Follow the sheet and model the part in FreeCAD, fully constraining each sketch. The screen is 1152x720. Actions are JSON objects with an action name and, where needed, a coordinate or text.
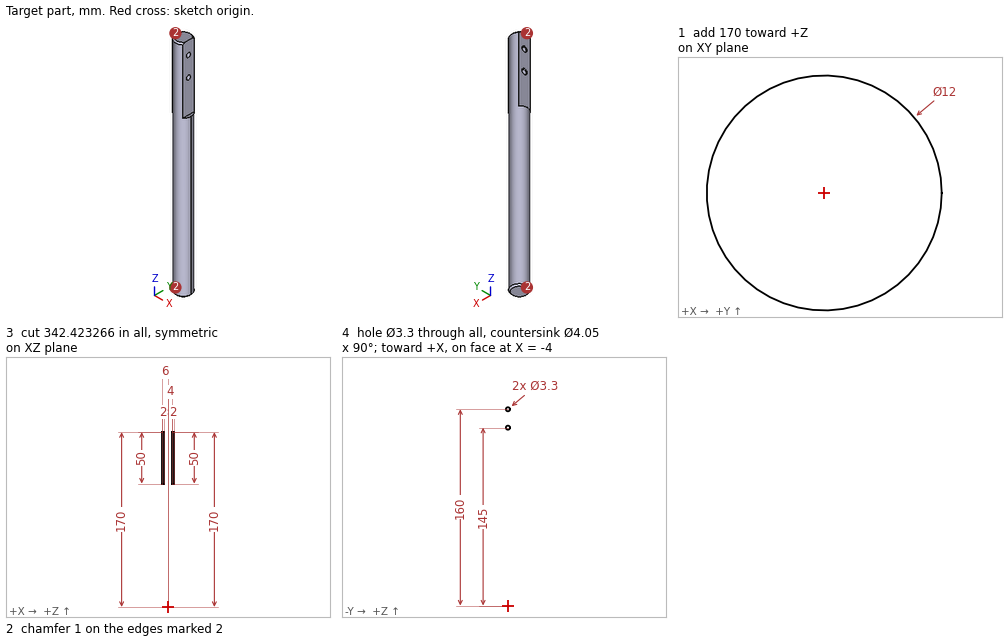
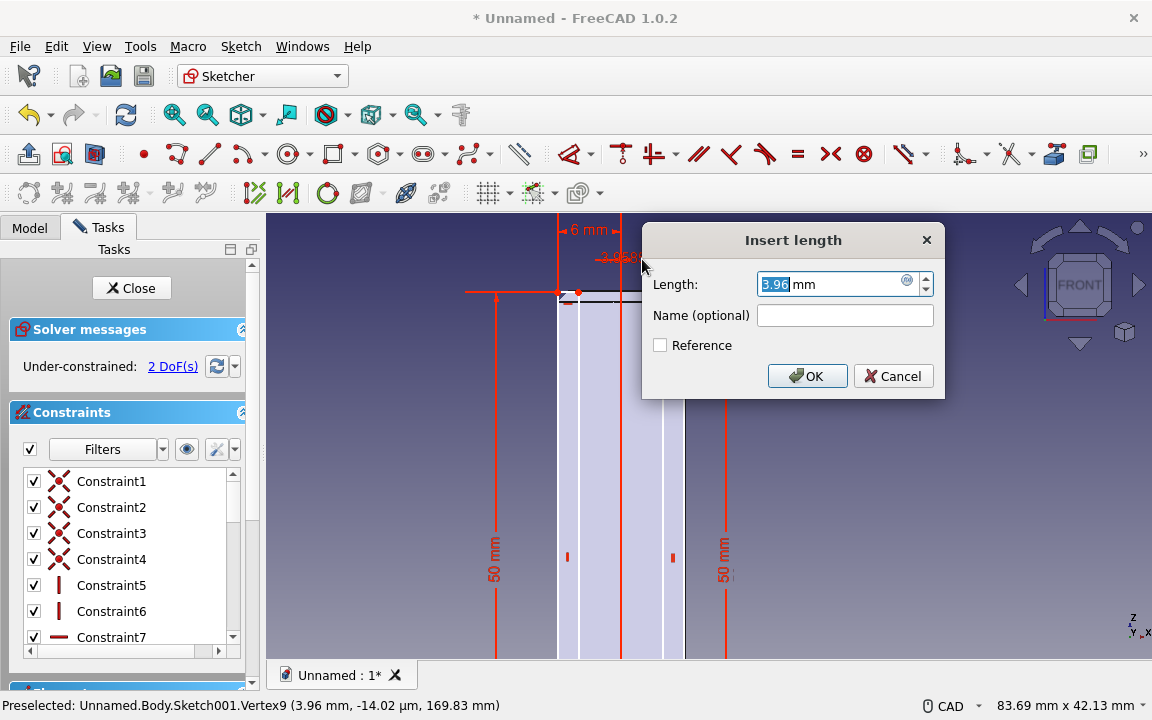
{"action": "type", "text": "4"}
{"action": "key", "text": "Return"}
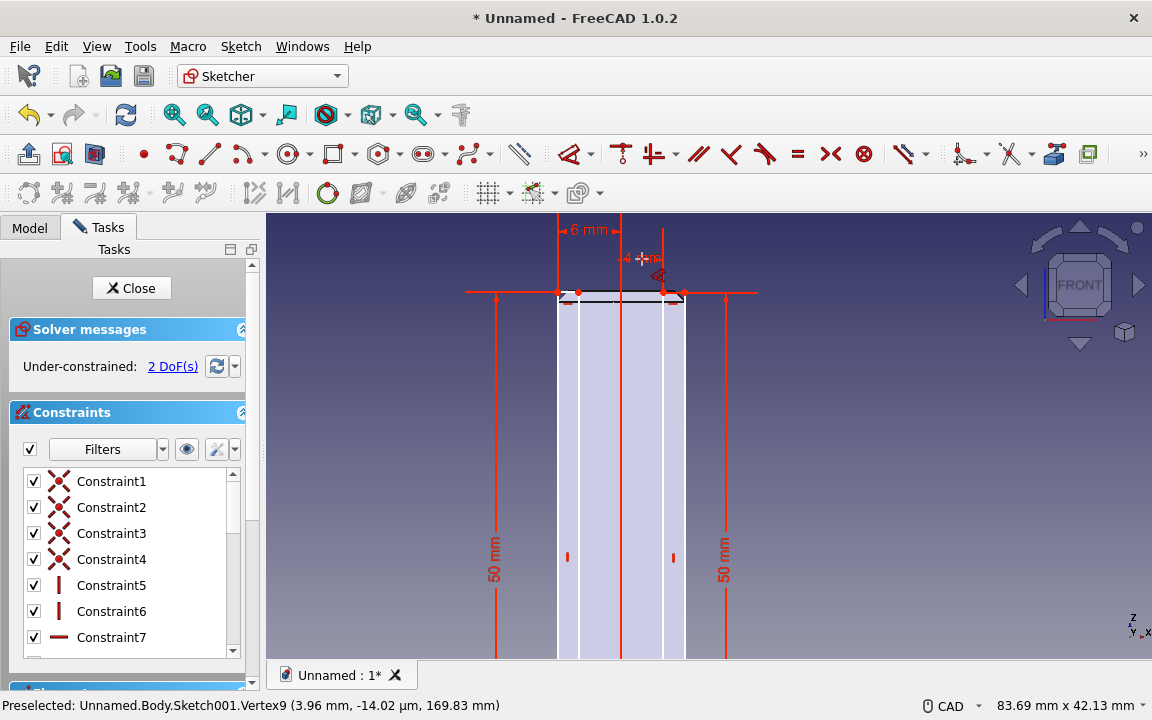
{"action": "left_click", "coordinate": [558, 292]}
{"action": "left_click", "coordinate": [524, 462]}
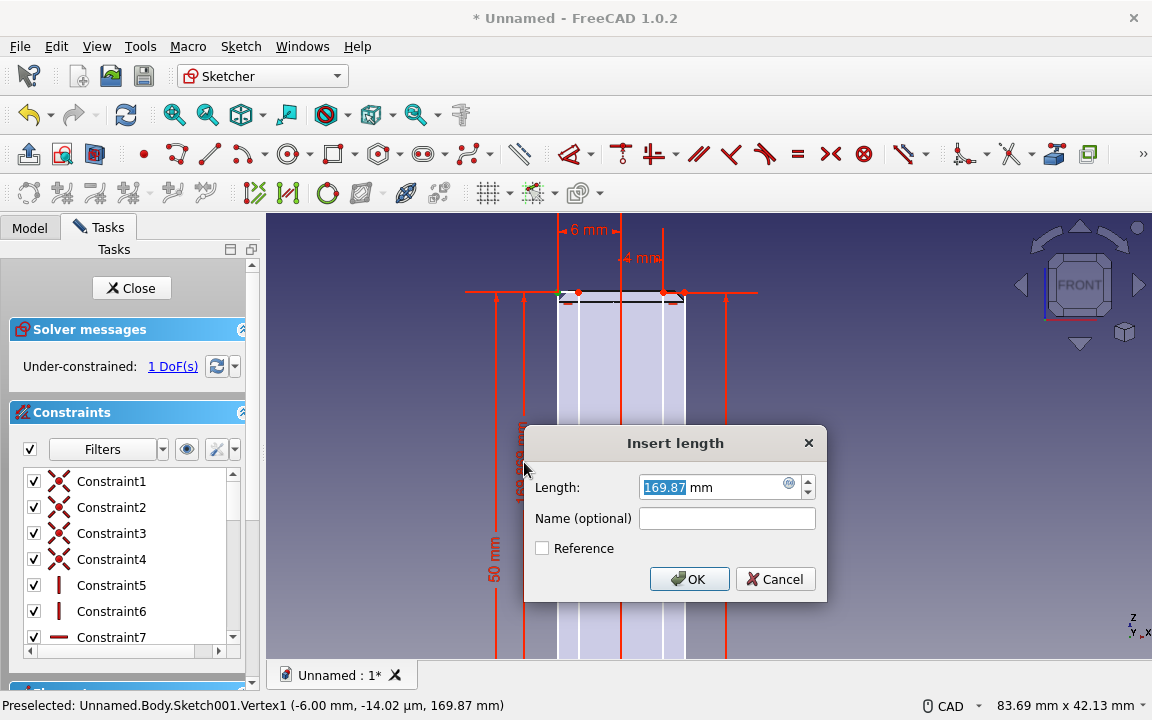
{"action": "type", "text": "170"}
{"action": "key", "text": "Return"}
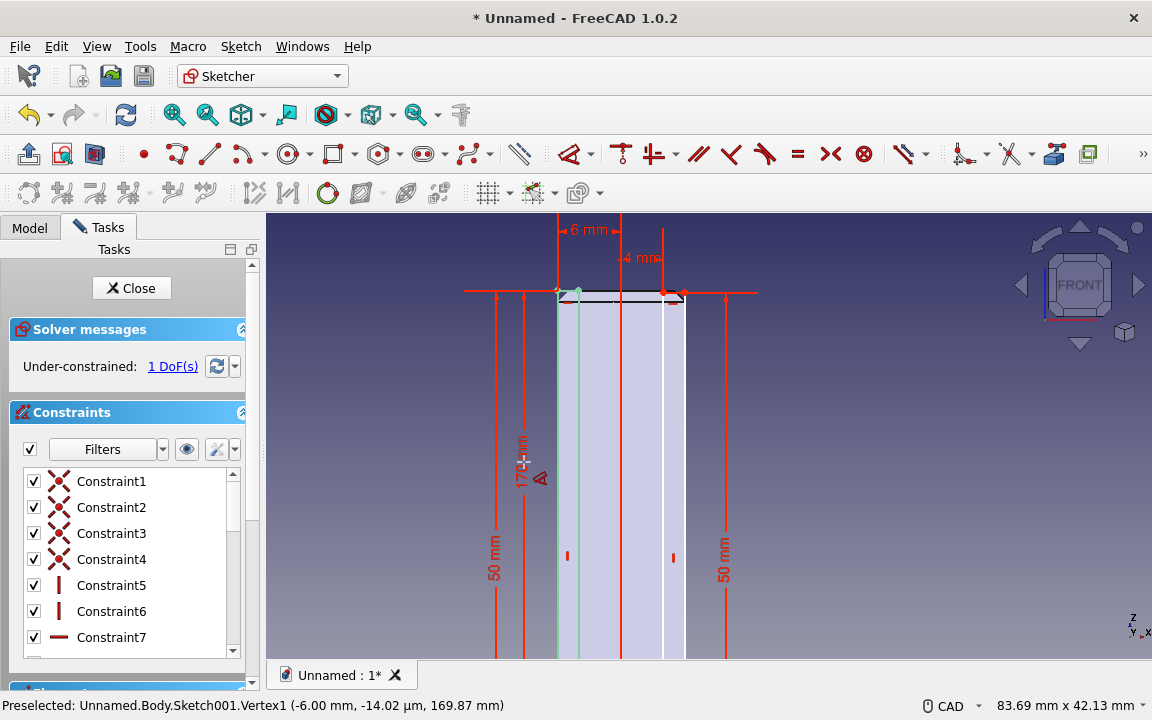
{"action": "left_click", "coordinate": [663, 293]}
{"action": "left_click", "coordinate": [721, 462]}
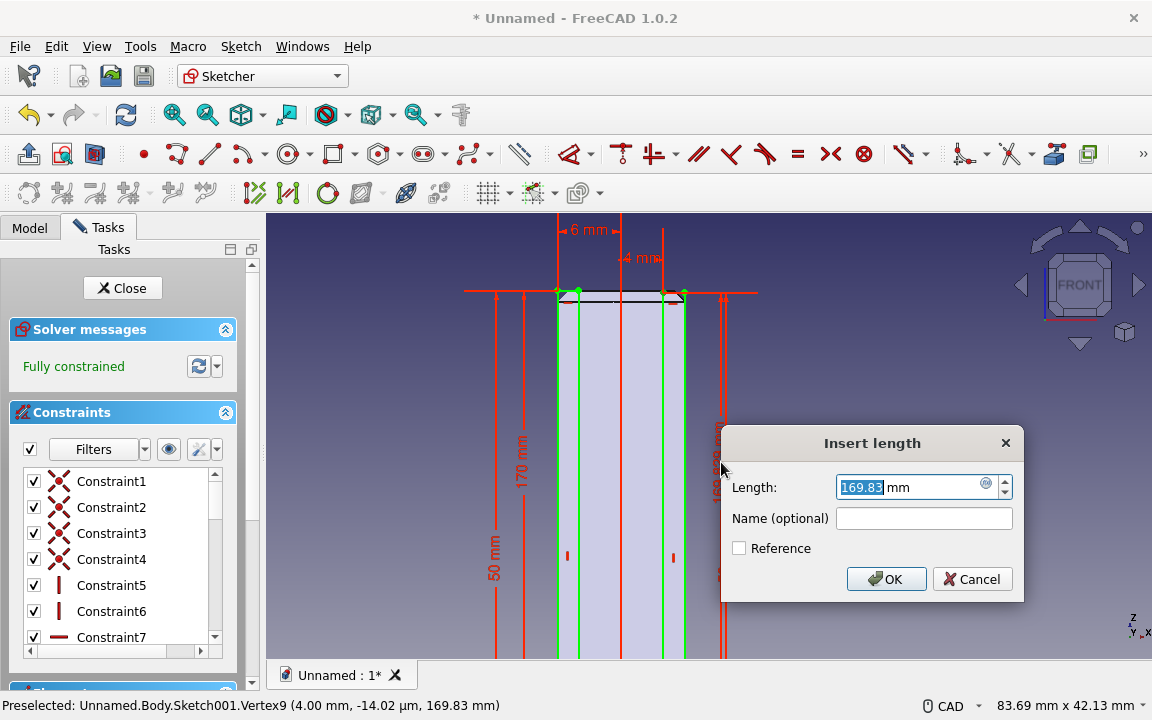
{"action": "type", "text": "170"}
{"action": "key", "text": "Return"}
{"action": "key", "text": "Escape"}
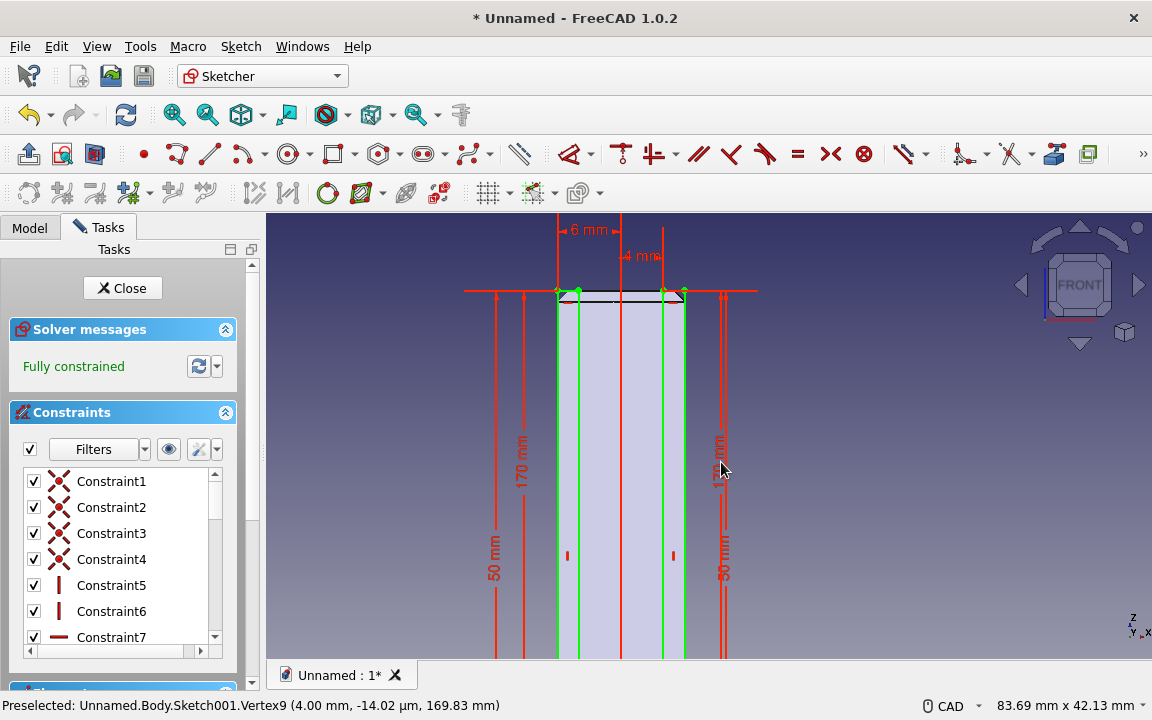
{"action": "left_click", "coordinate": [123, 288]}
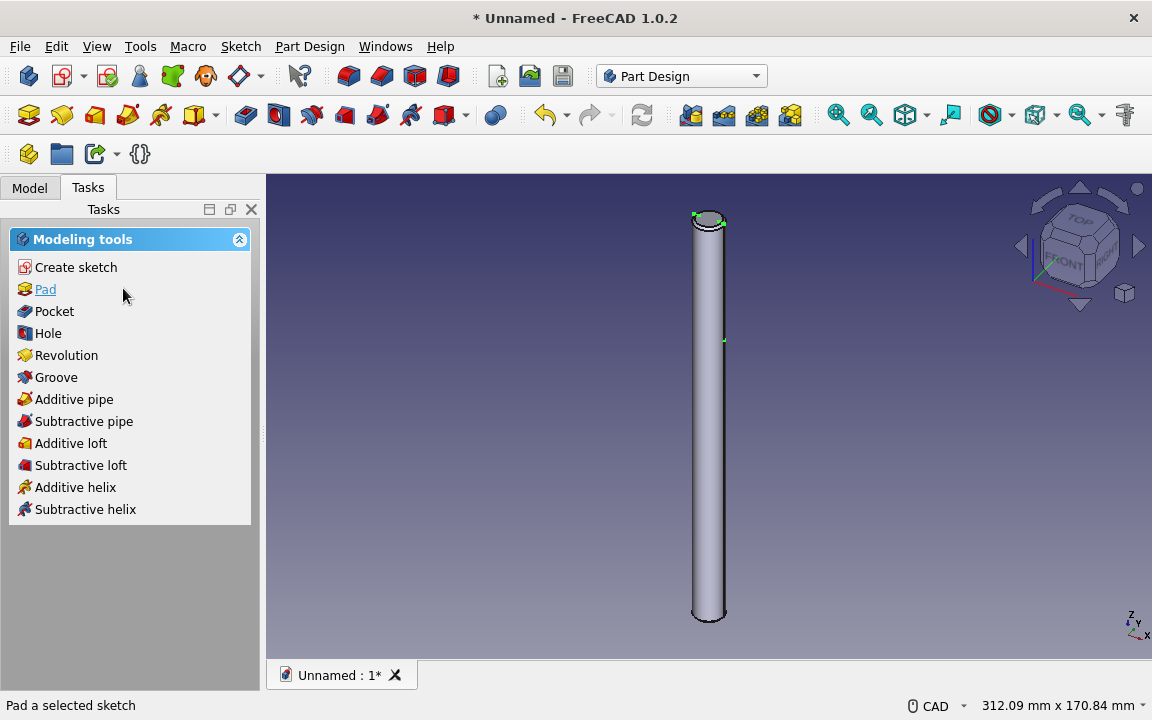
{"action": "left_click", "coordinate": [246, 116]}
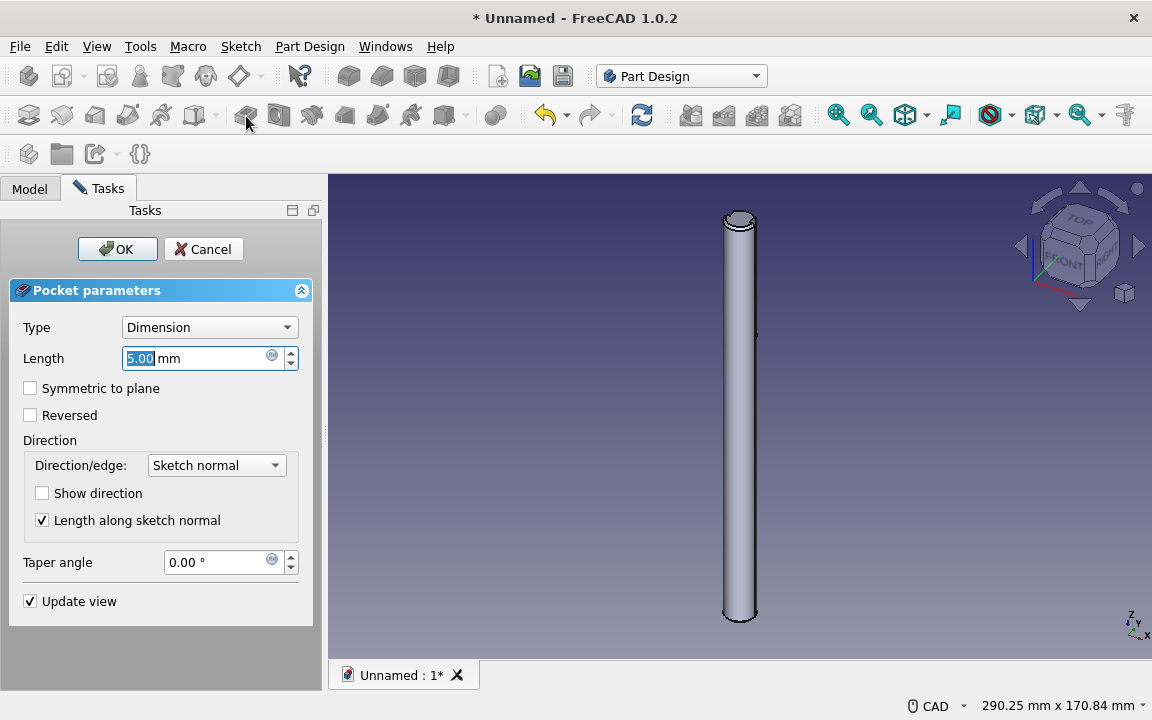
{"action": "type", "text": "342.423266"}
{"action": "key", "text": "Tab"}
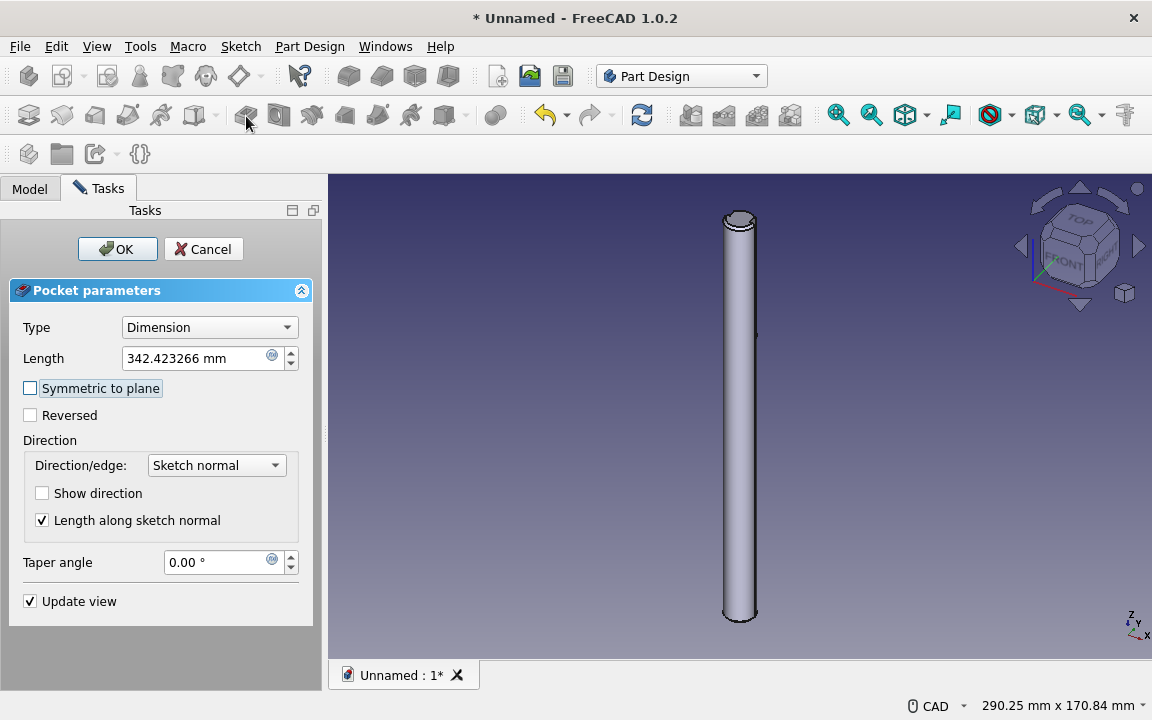
{"action": "left_click", "coordinate": [31, 388]}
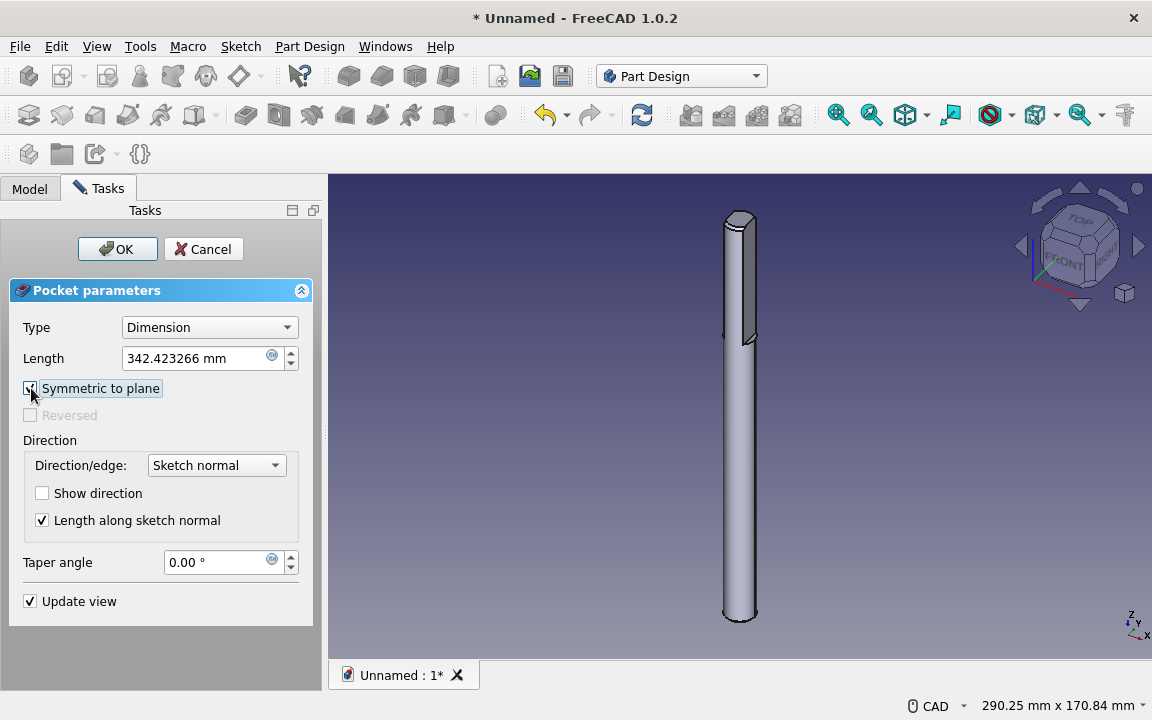
{"action": "left_click", "coordinate": [118, 249]}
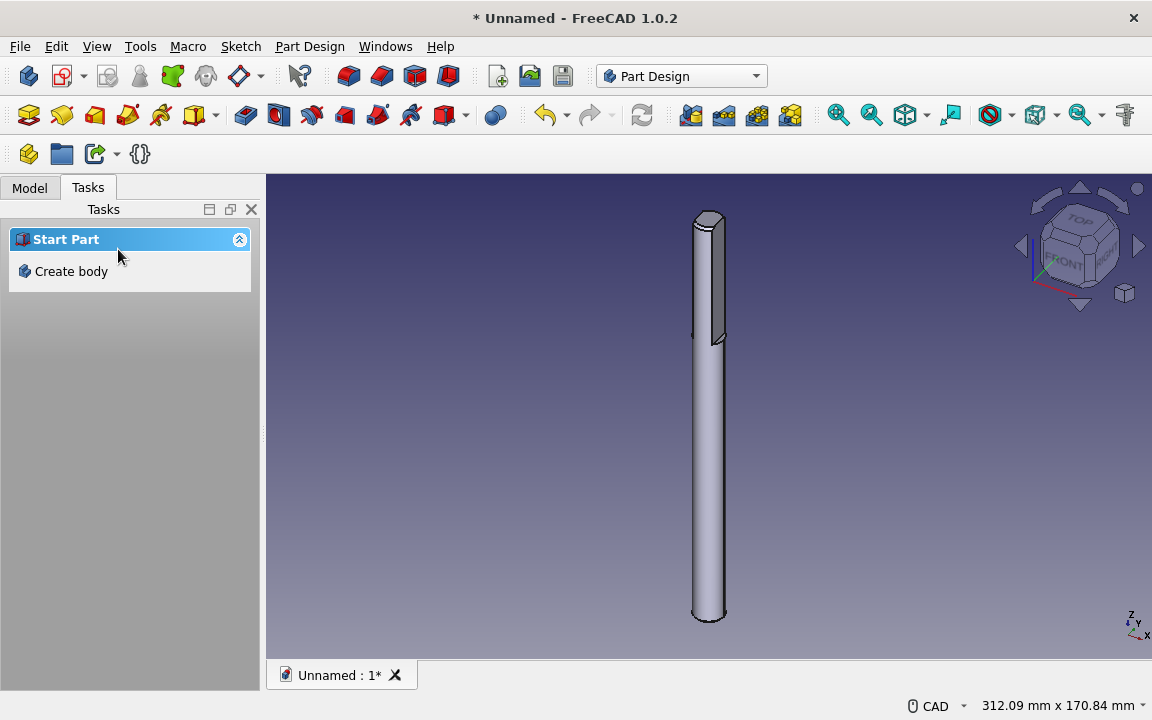
{"action": "key", "text": "6"}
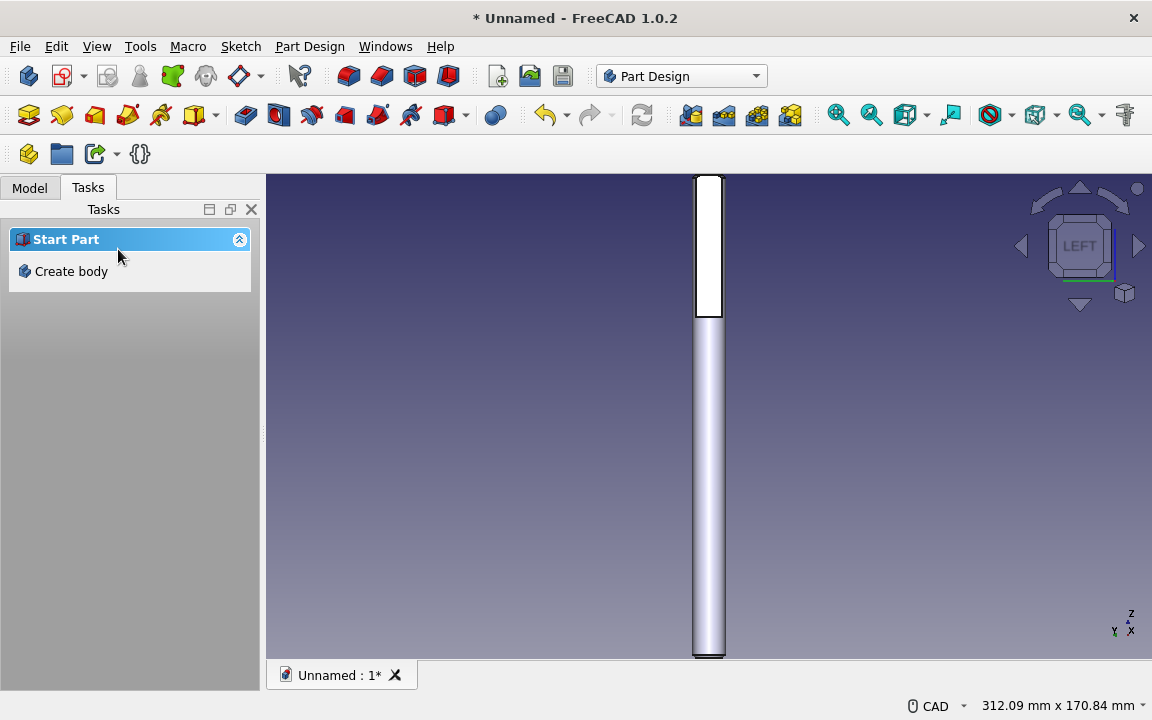
{"action": "left_click", "coordinate": [709, 205]}